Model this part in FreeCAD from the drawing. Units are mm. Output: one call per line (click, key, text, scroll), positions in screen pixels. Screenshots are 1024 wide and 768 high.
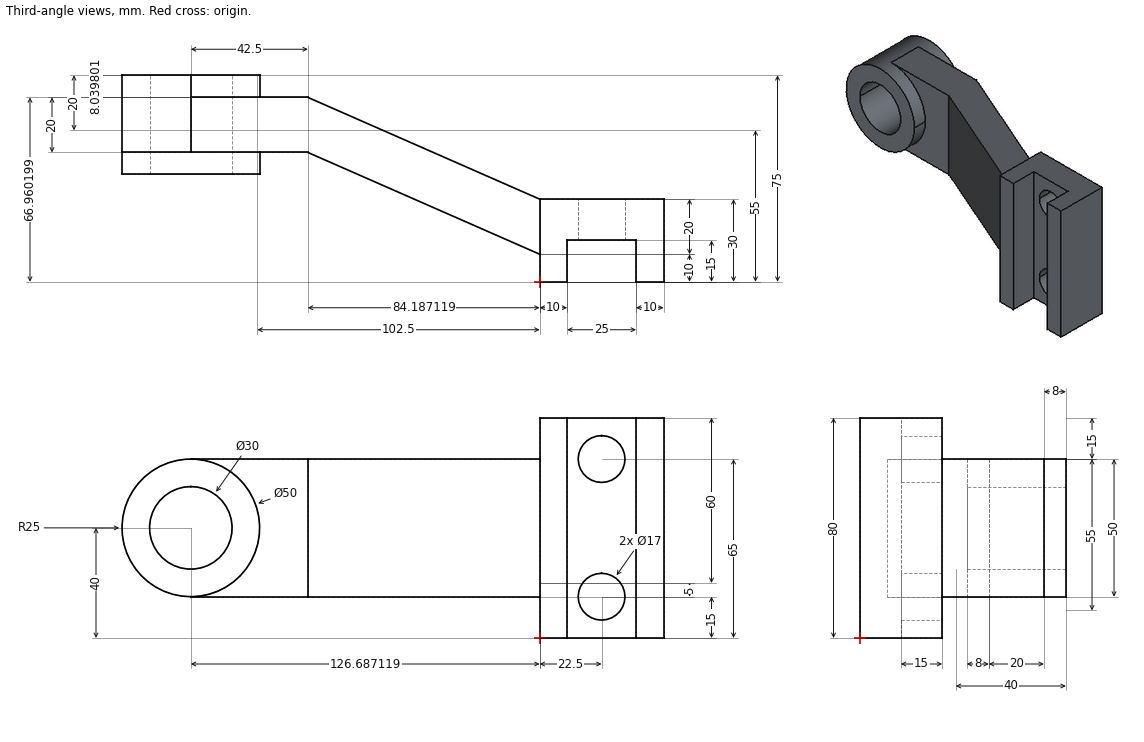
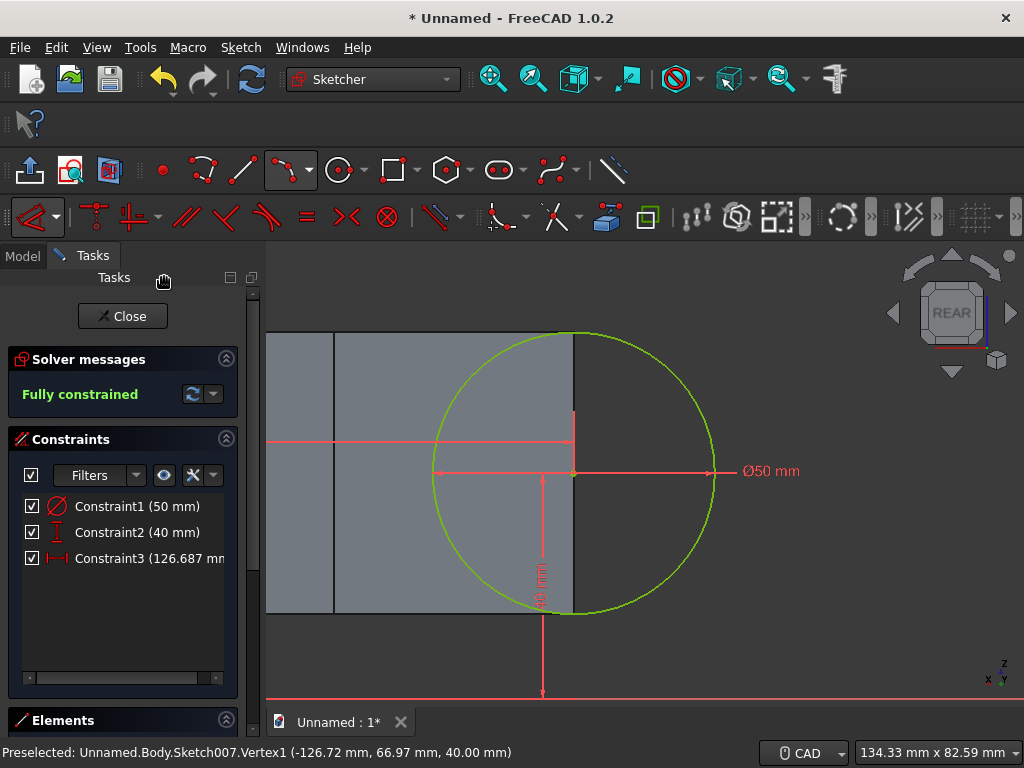
click(123, 316)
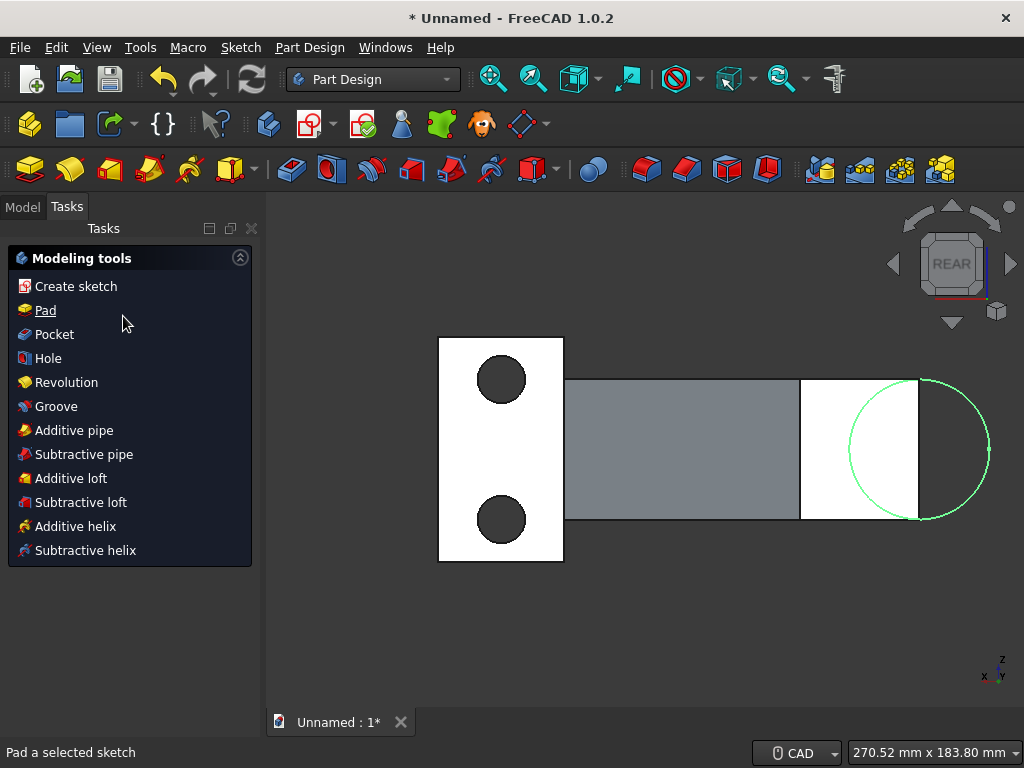
click(30, 170)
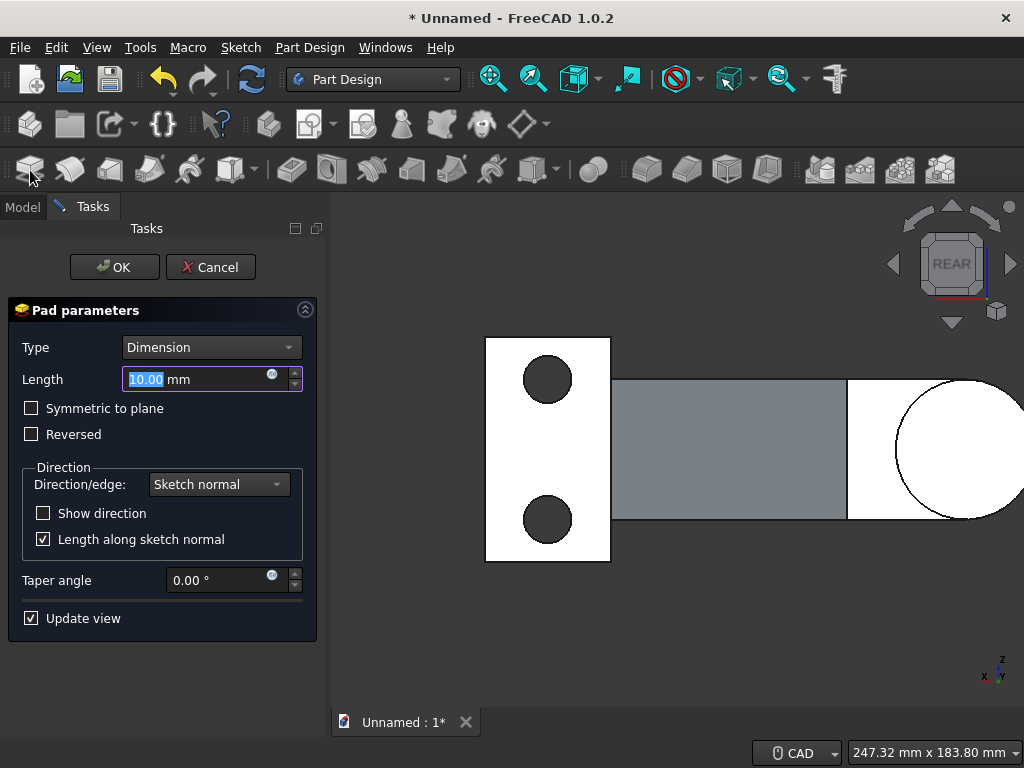
text(8)
key(Tab)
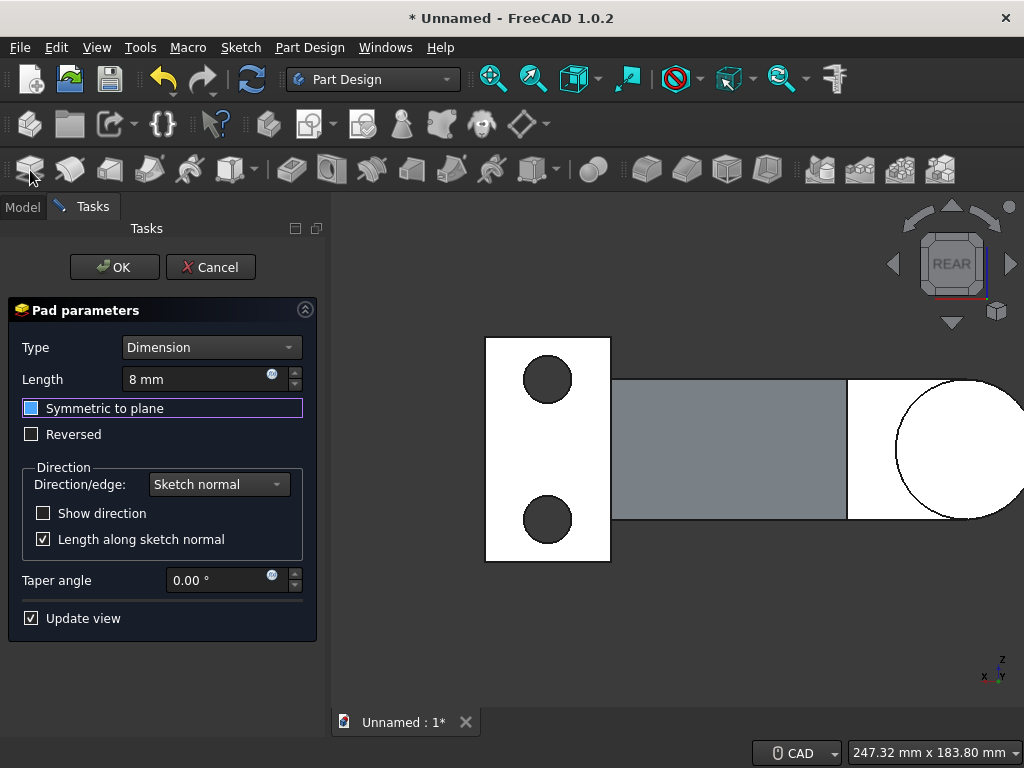
click(115, 267)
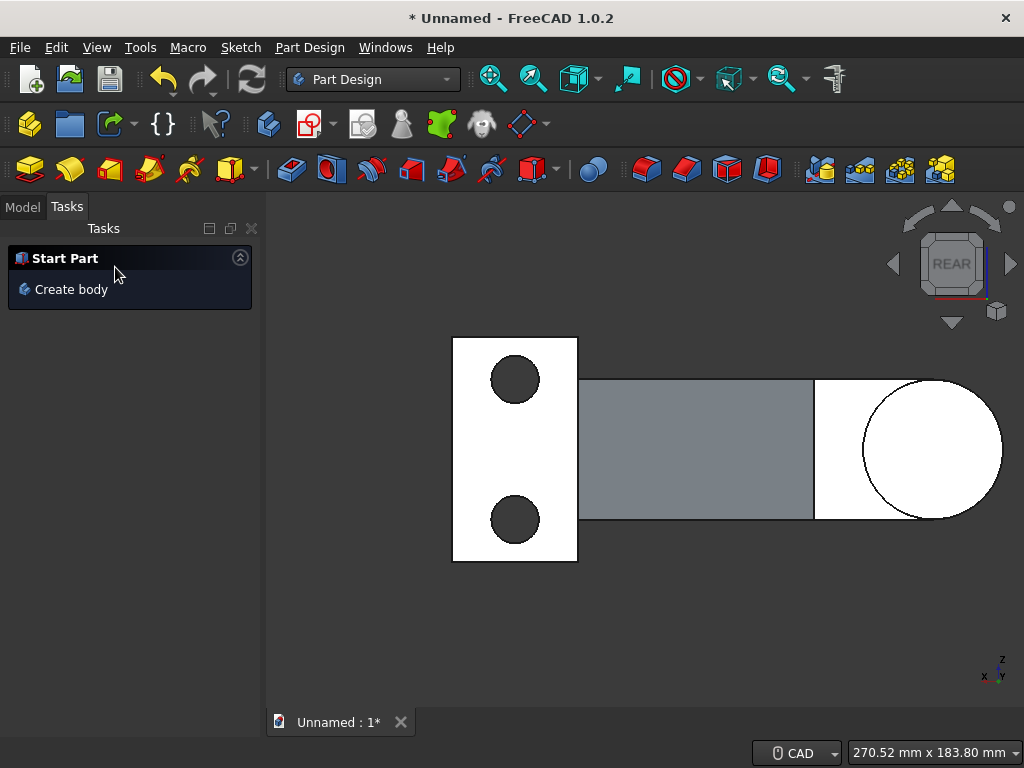
key(0)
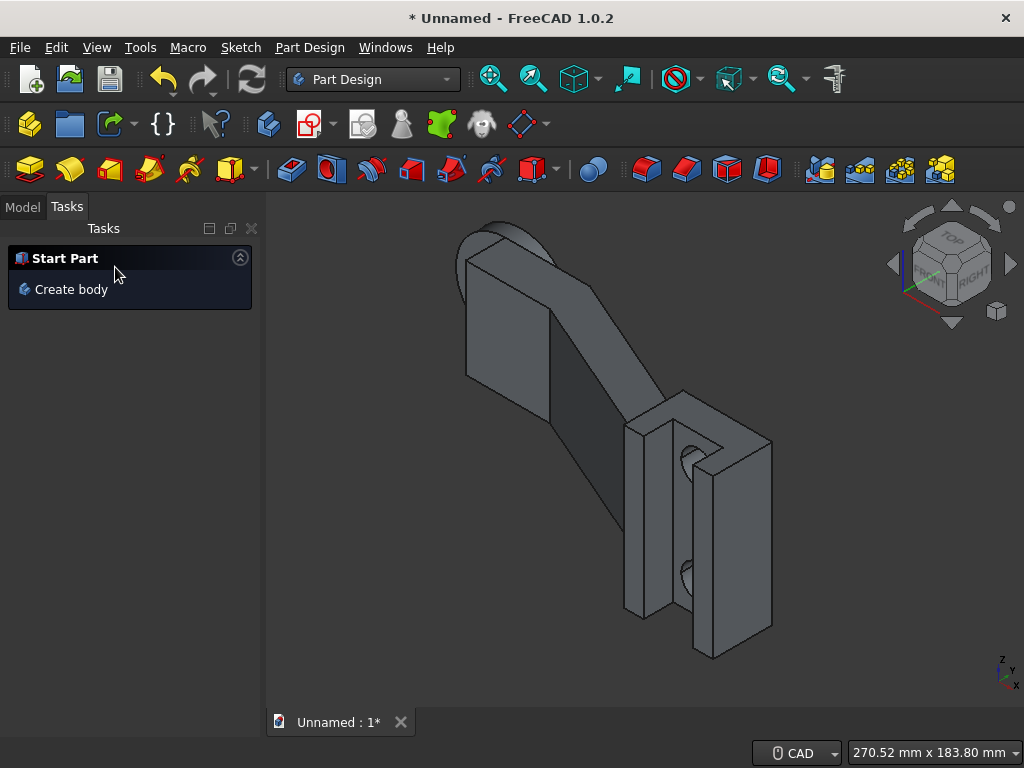
click(494, 80)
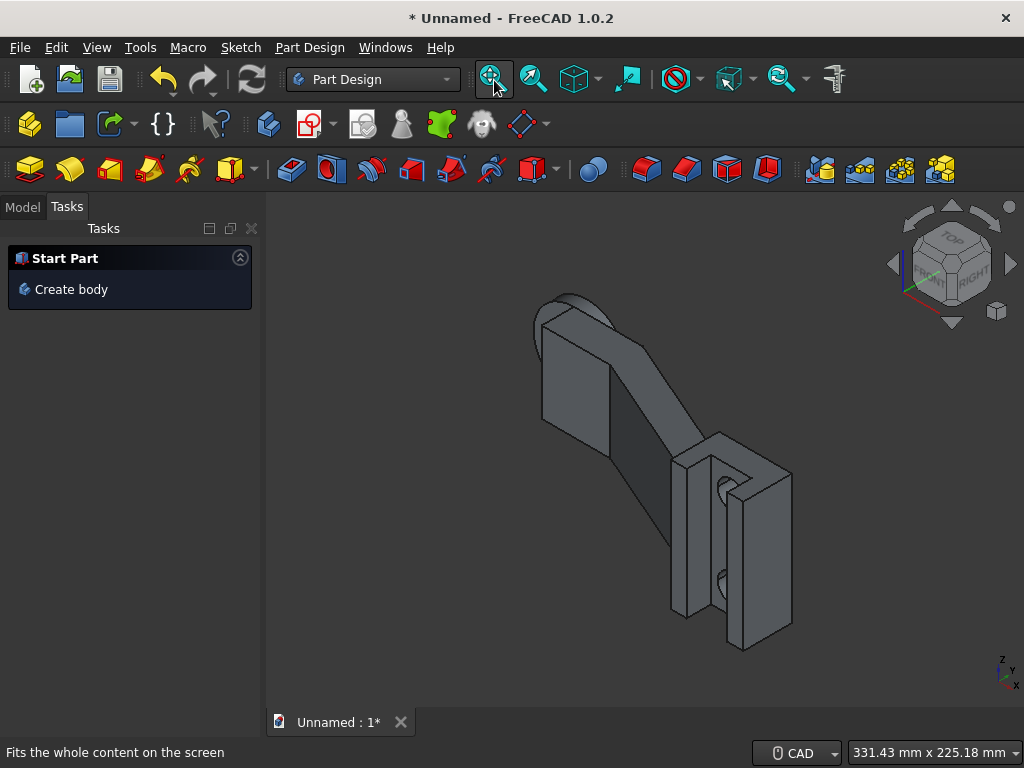
click(576, 391)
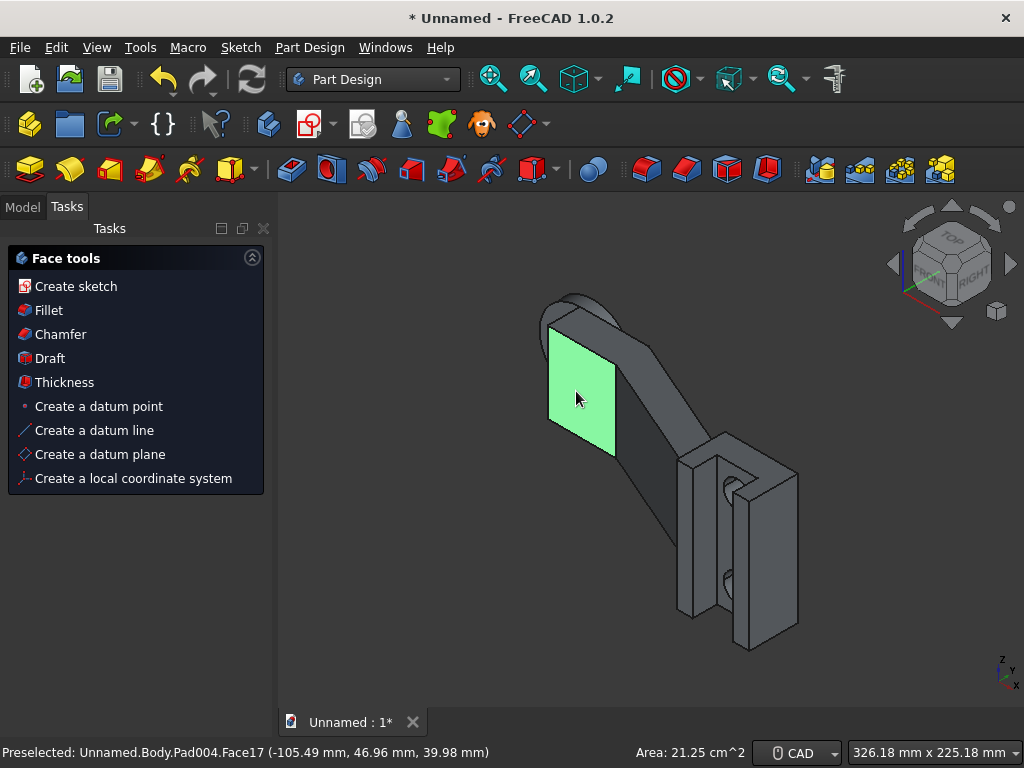
click(310, 124)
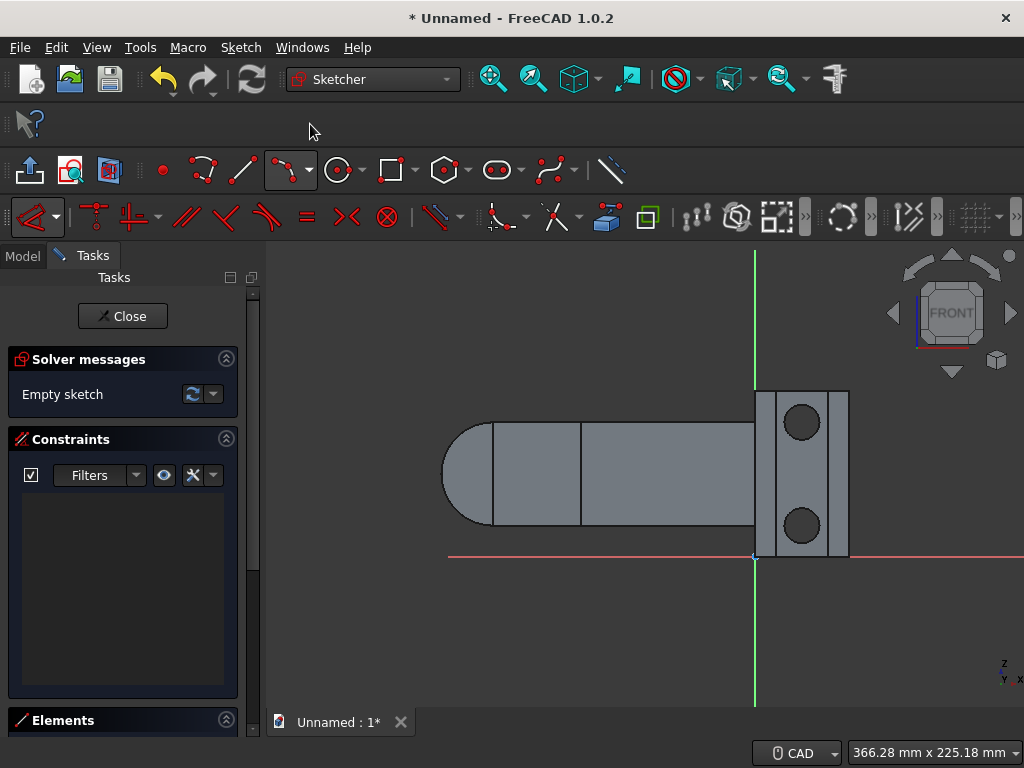
scroll(404, 474, up, 5)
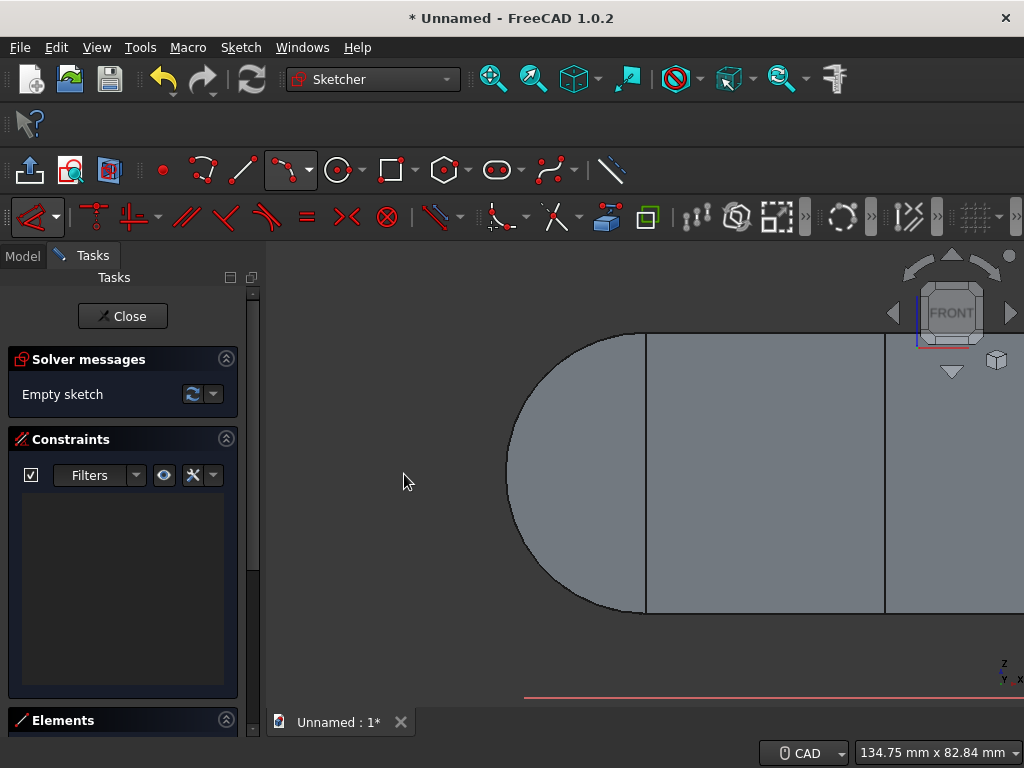
key(g)
key(l)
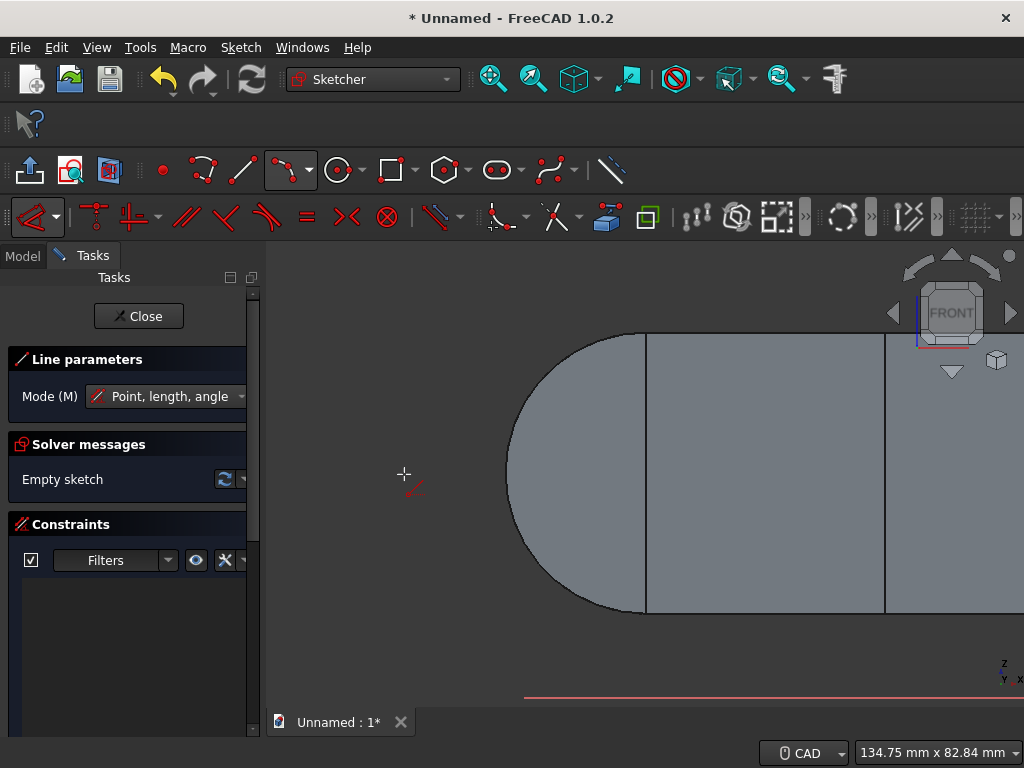
click(646, 614)
click(646, 333)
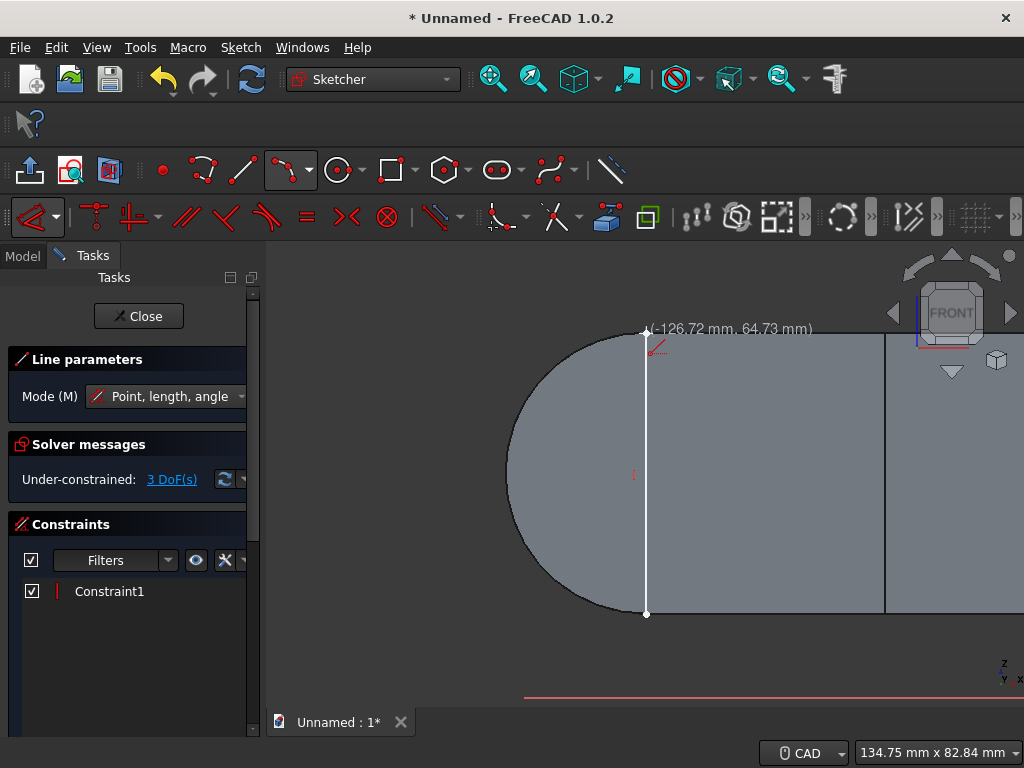
key(g)
key(3)
key(a)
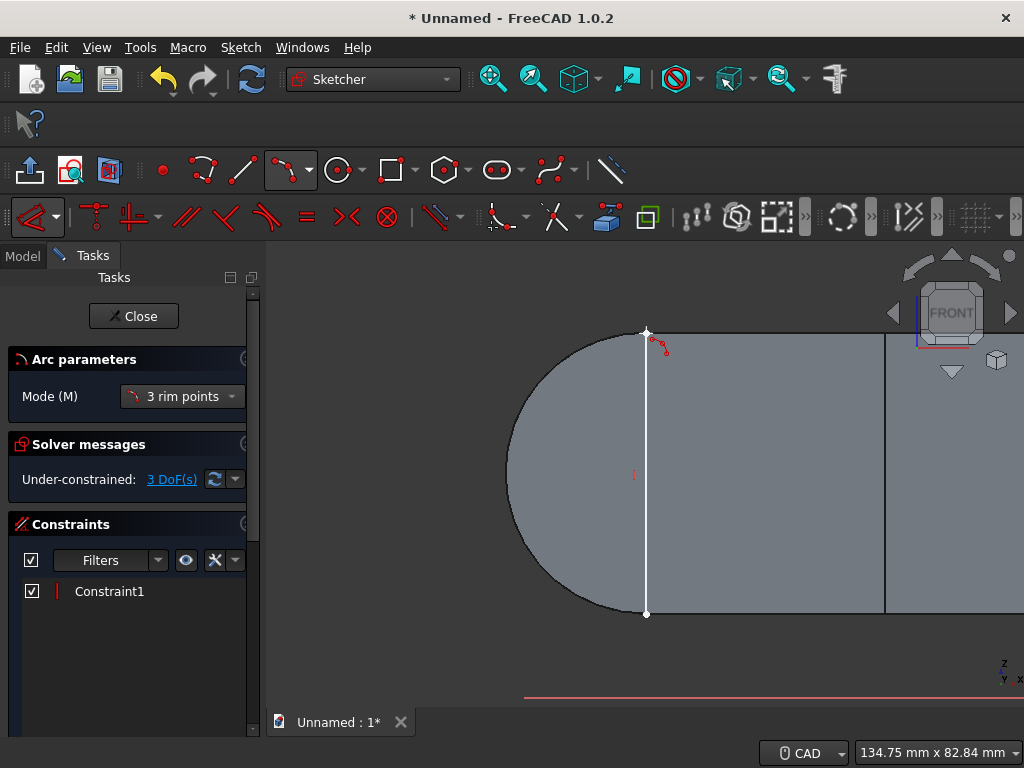
click(646, 334)
click(646, 615)
click(506, 473)
key(Escape)